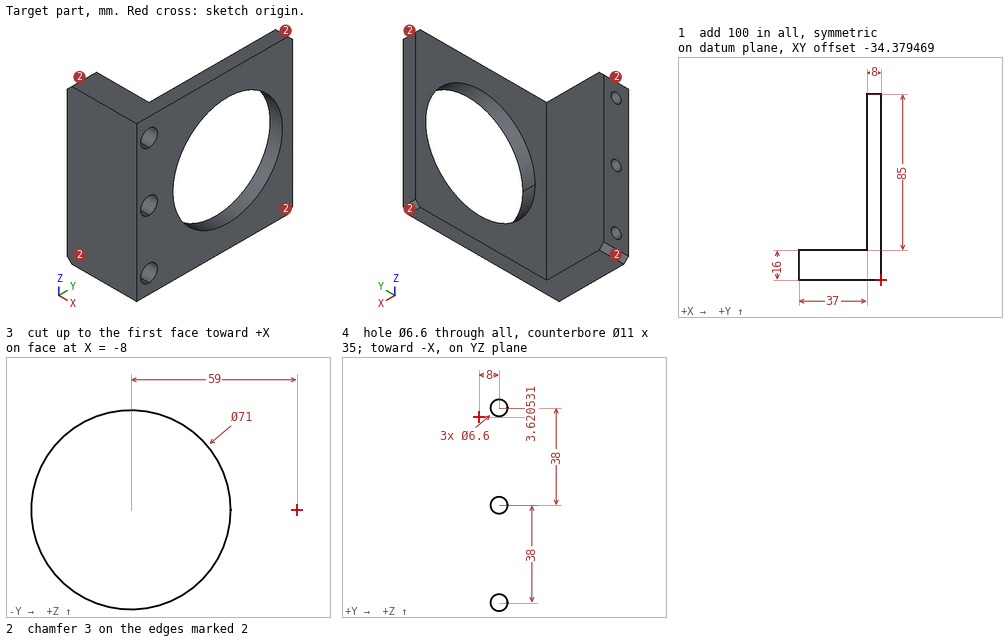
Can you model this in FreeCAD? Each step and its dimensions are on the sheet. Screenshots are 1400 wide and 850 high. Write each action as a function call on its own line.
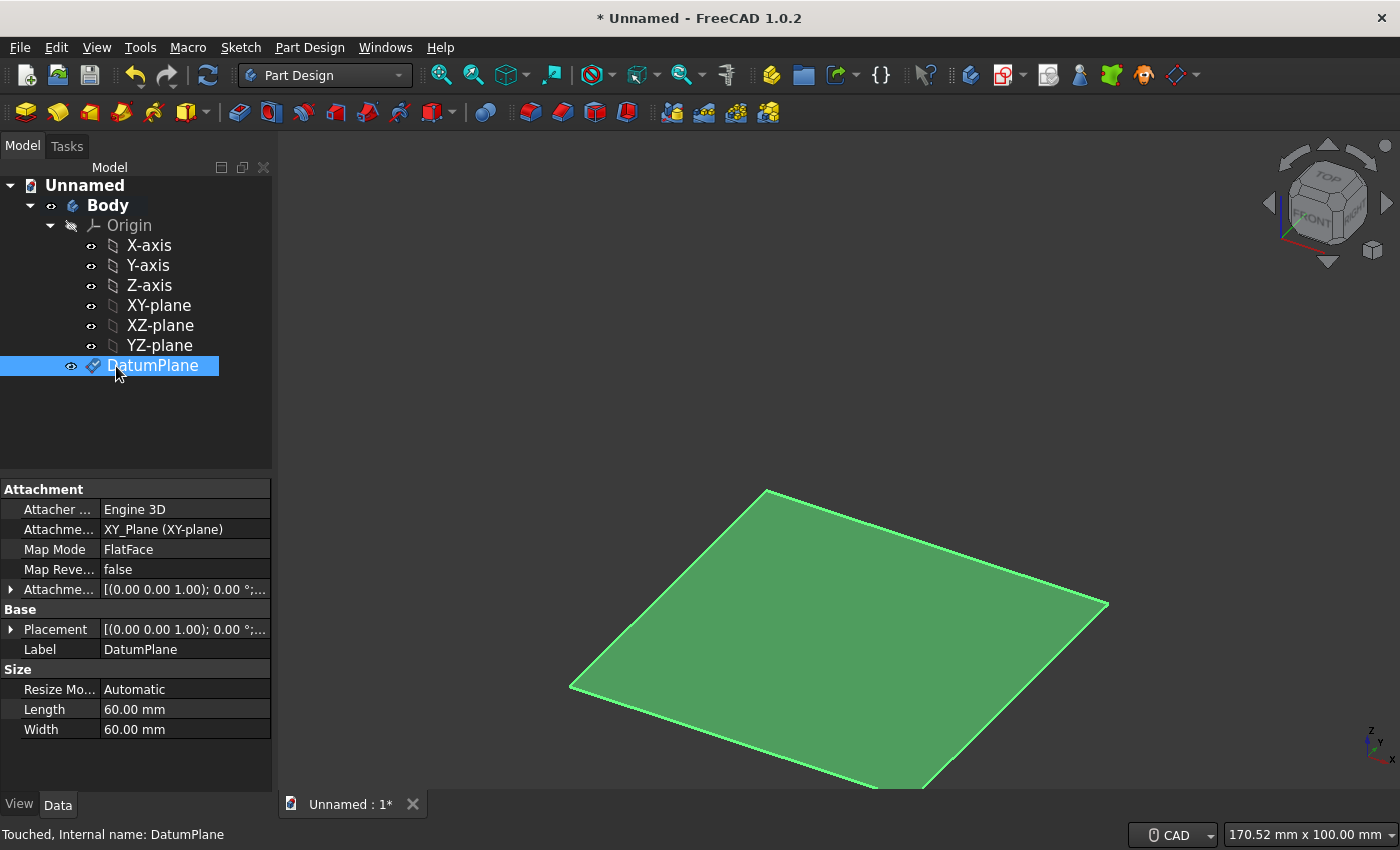
click(1004, 76)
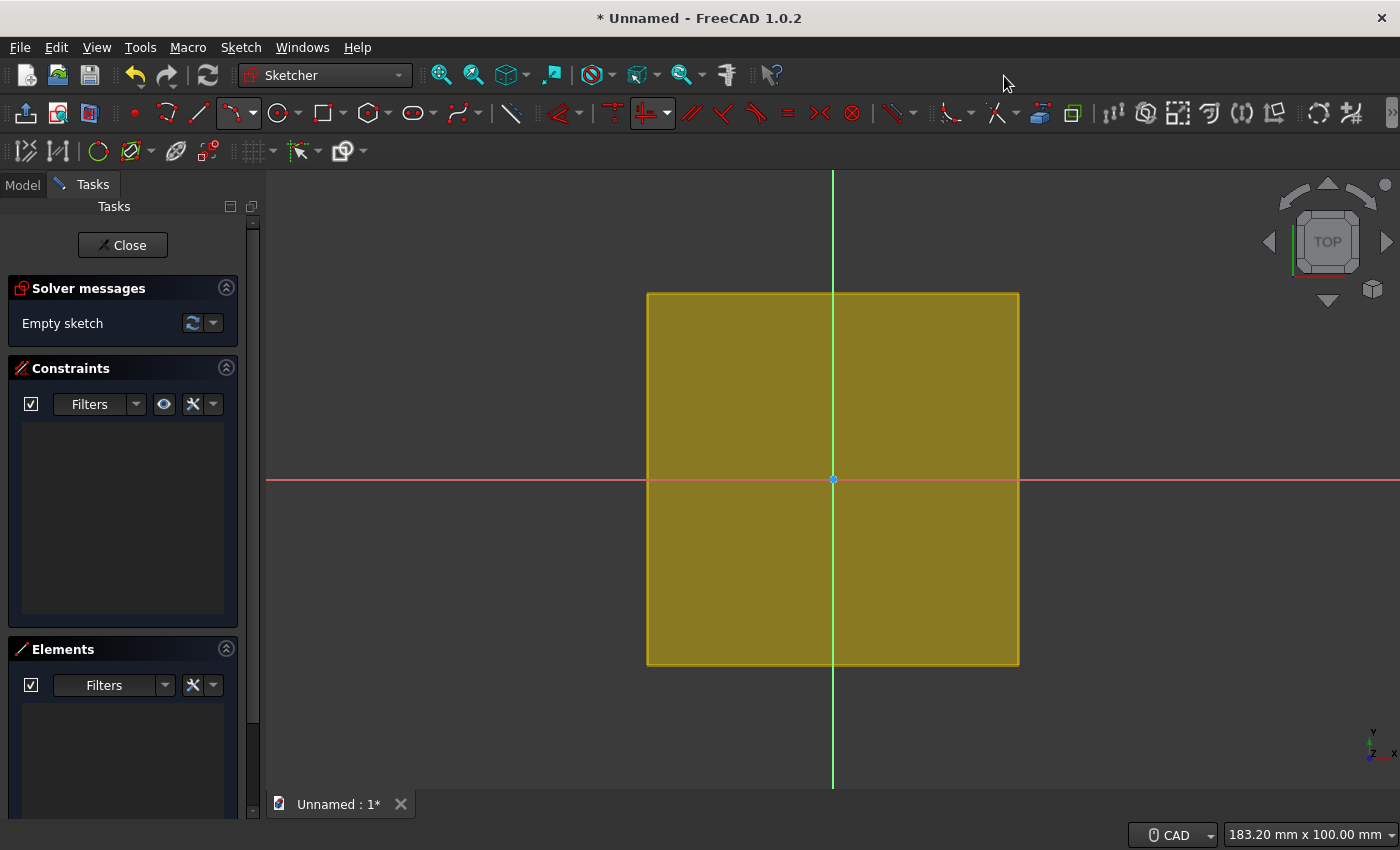
scroll(851, 761, down, 3)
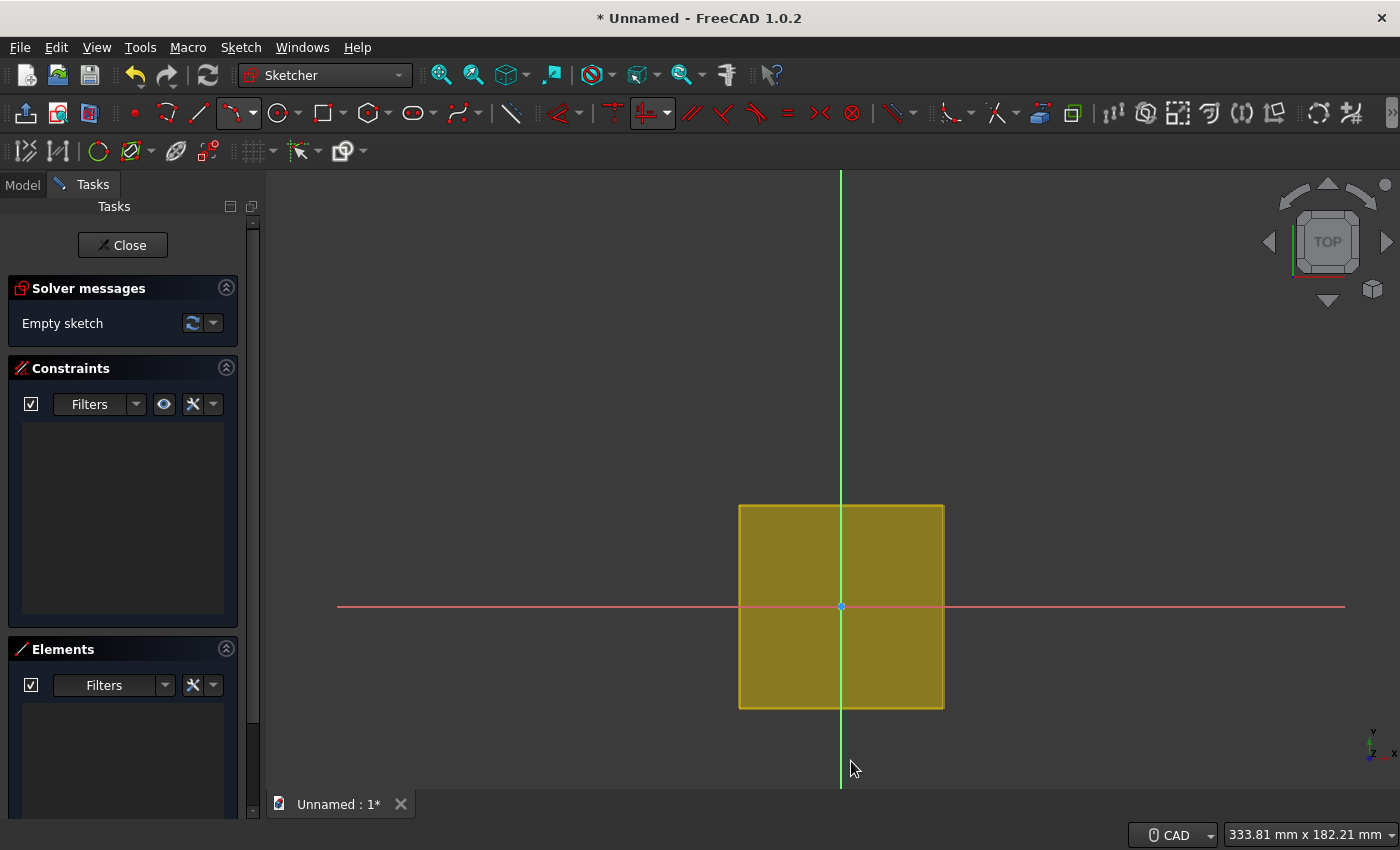
click(168, 114)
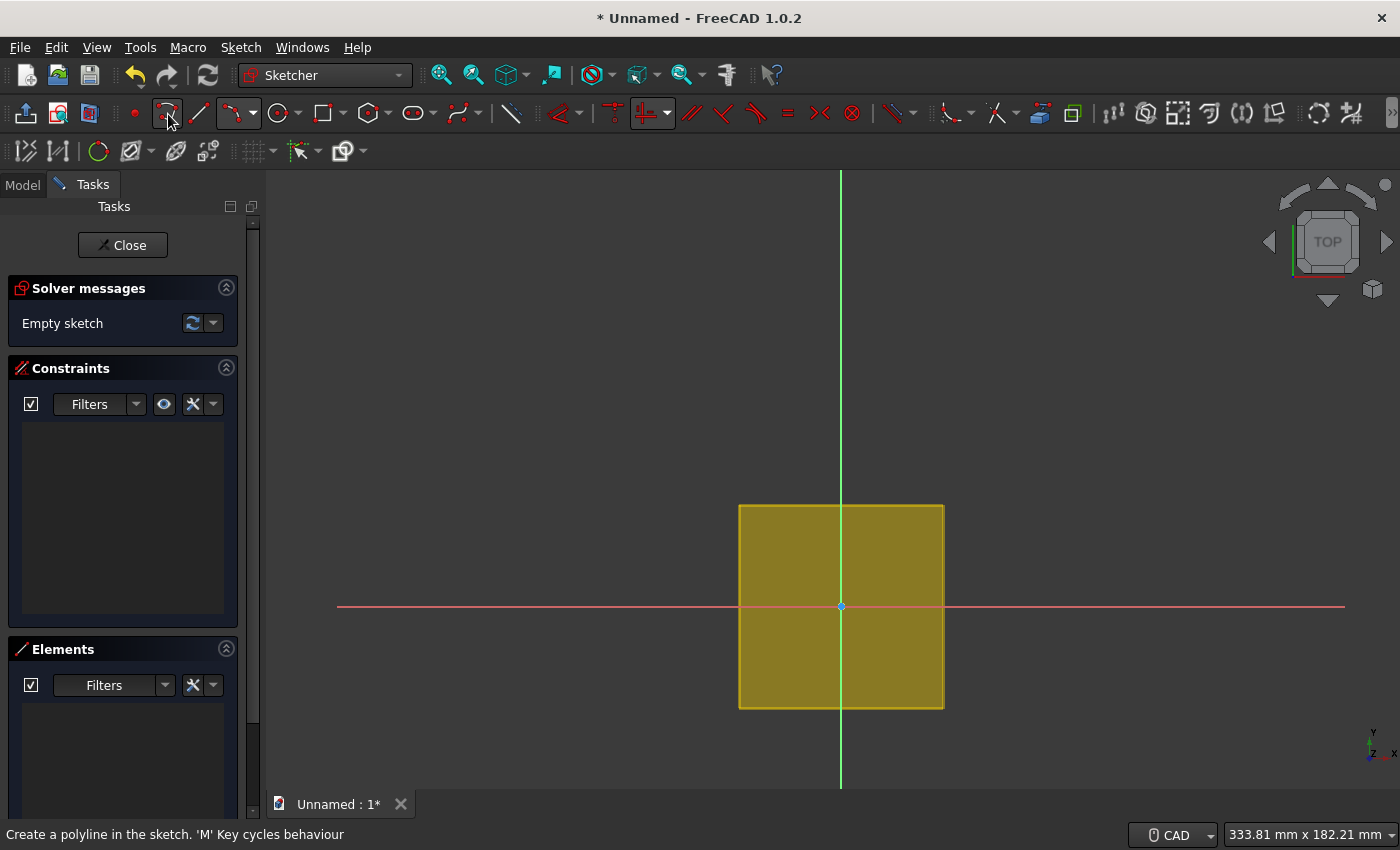
click(841, 607)
click(832, 264)
click(814, 264)
click(814, 553)
click(688, 553)
click(688, 598)
click(841, 607)
key(Escape)
key(Escape)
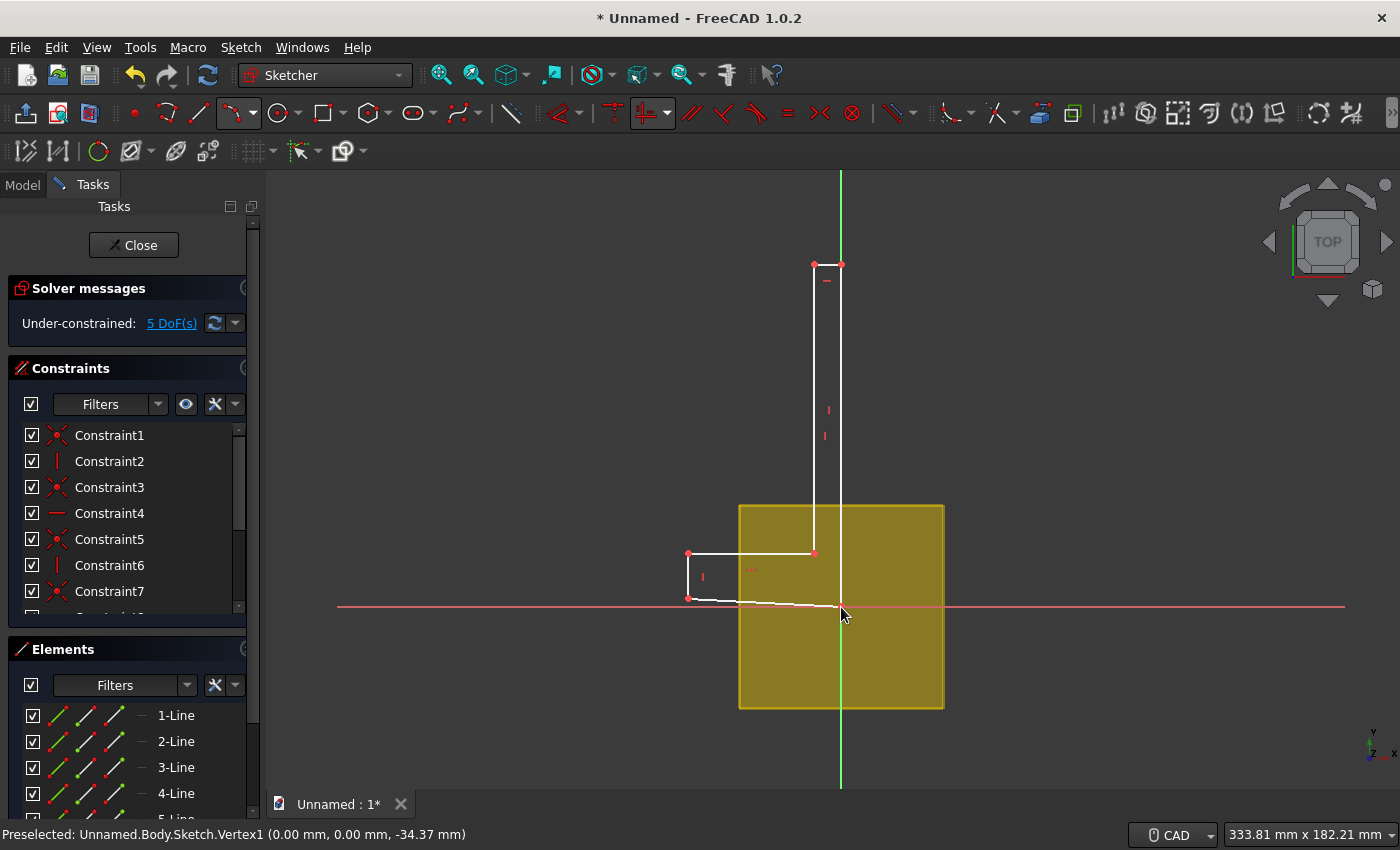
click(795, 605)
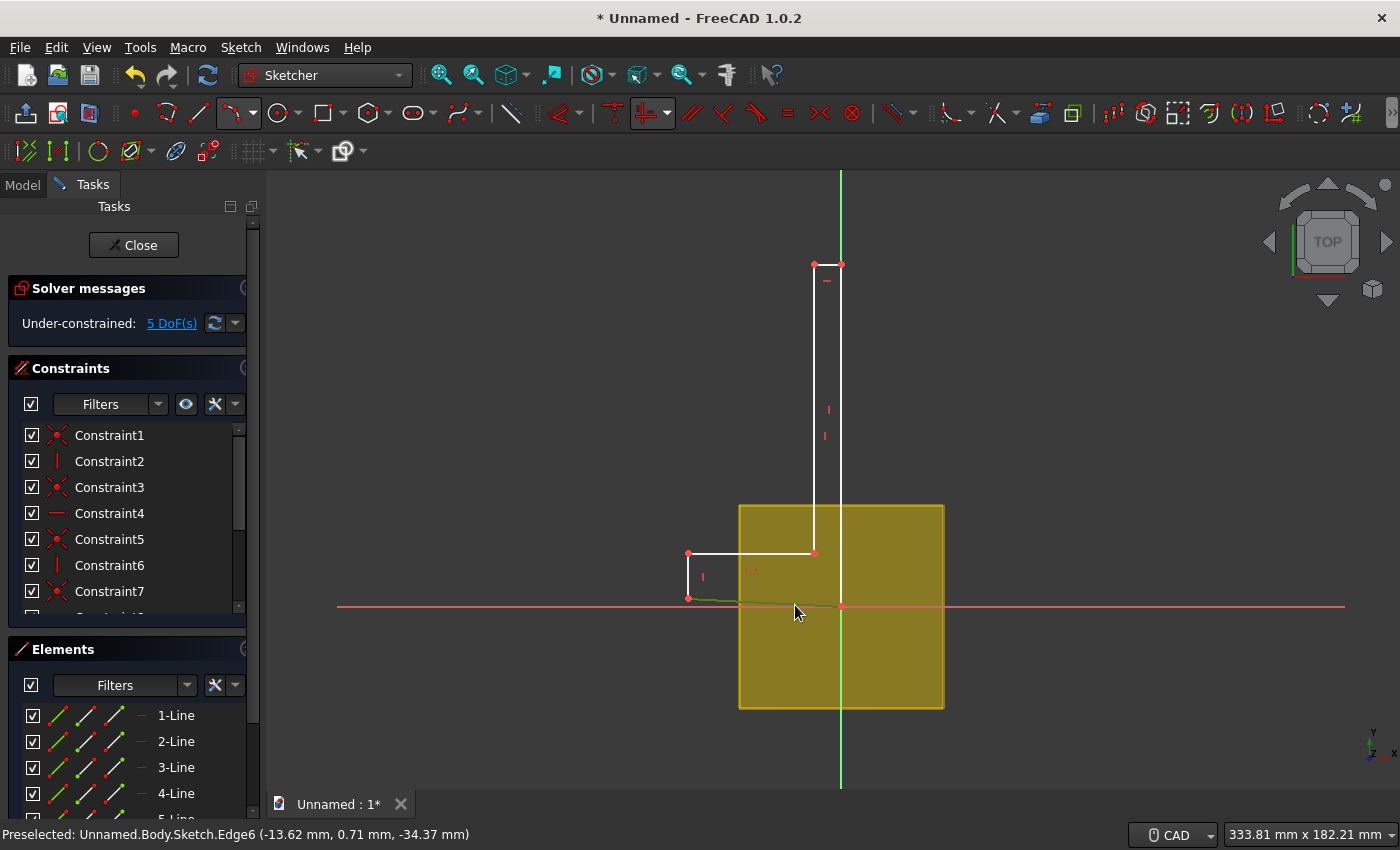
click(670, 114)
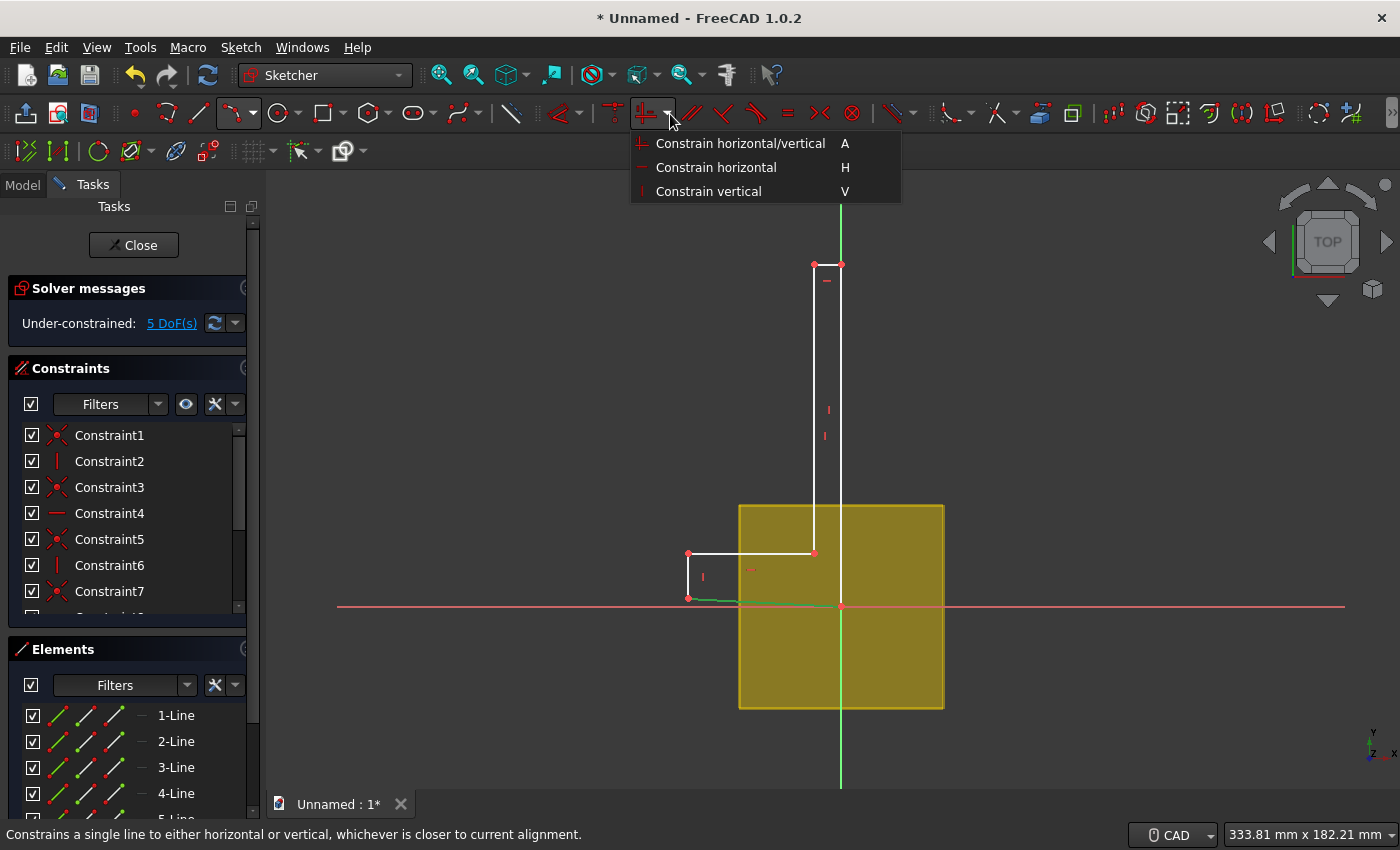
click(766, 167)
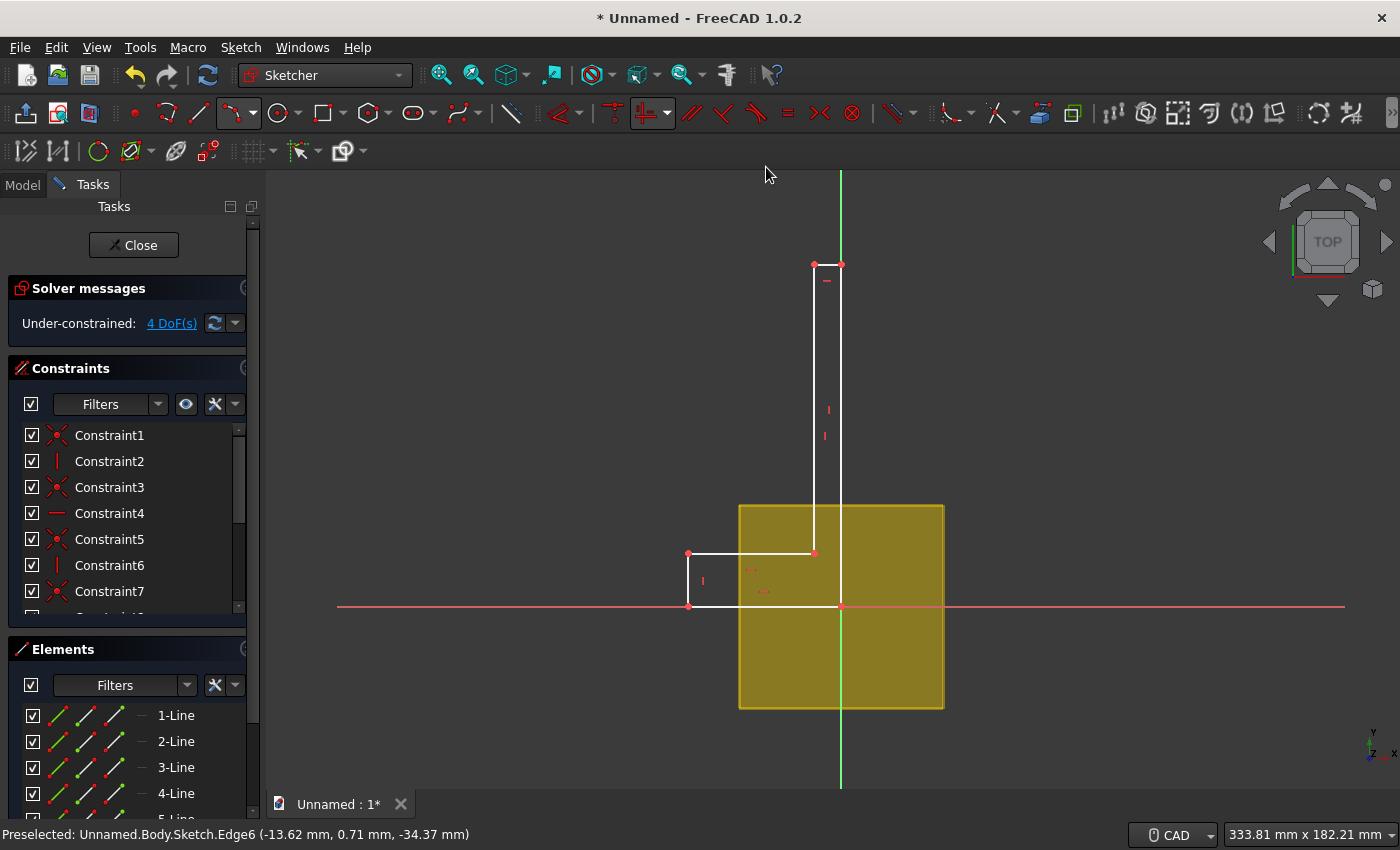
click(558, 114)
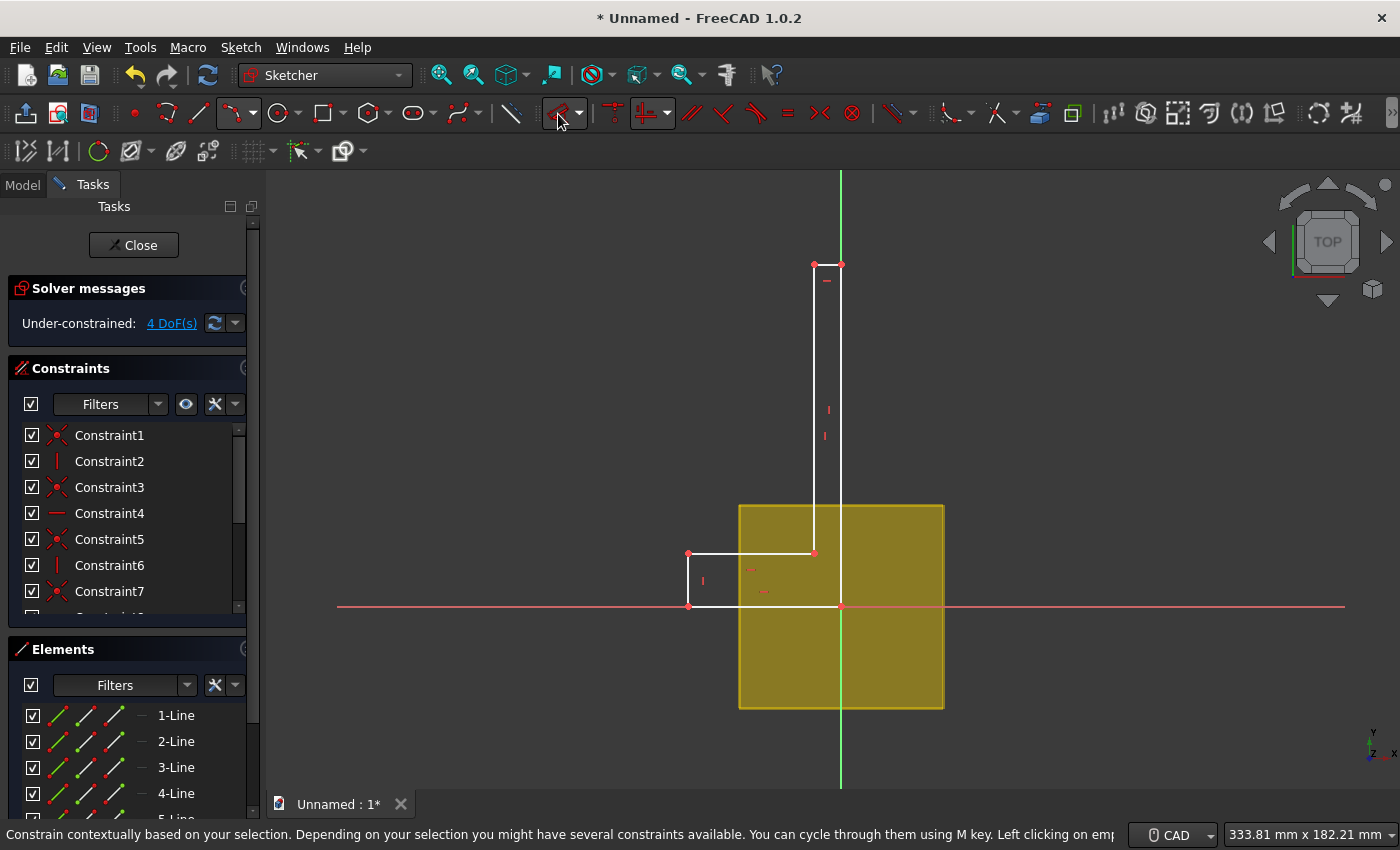
scroll(830, 265, up, 2)